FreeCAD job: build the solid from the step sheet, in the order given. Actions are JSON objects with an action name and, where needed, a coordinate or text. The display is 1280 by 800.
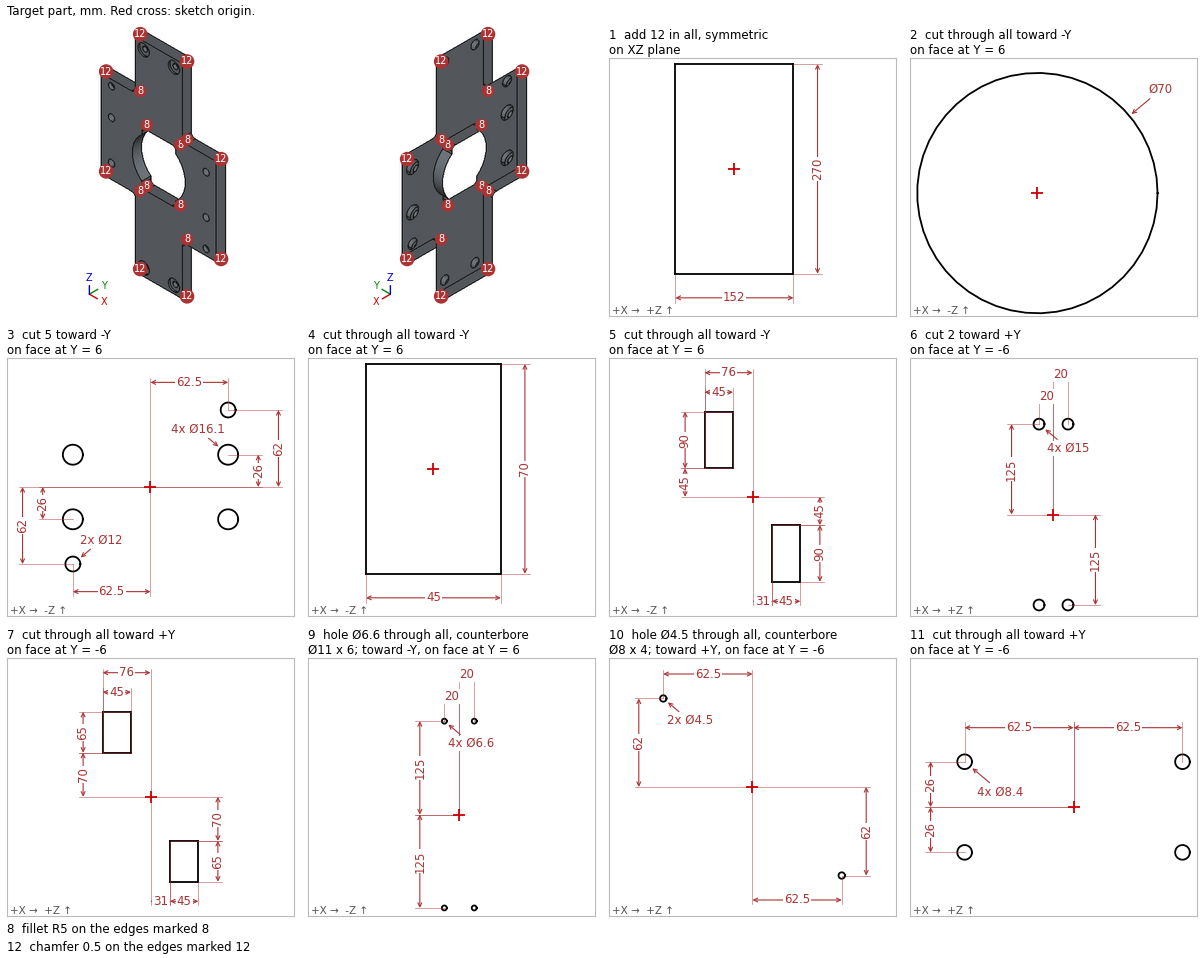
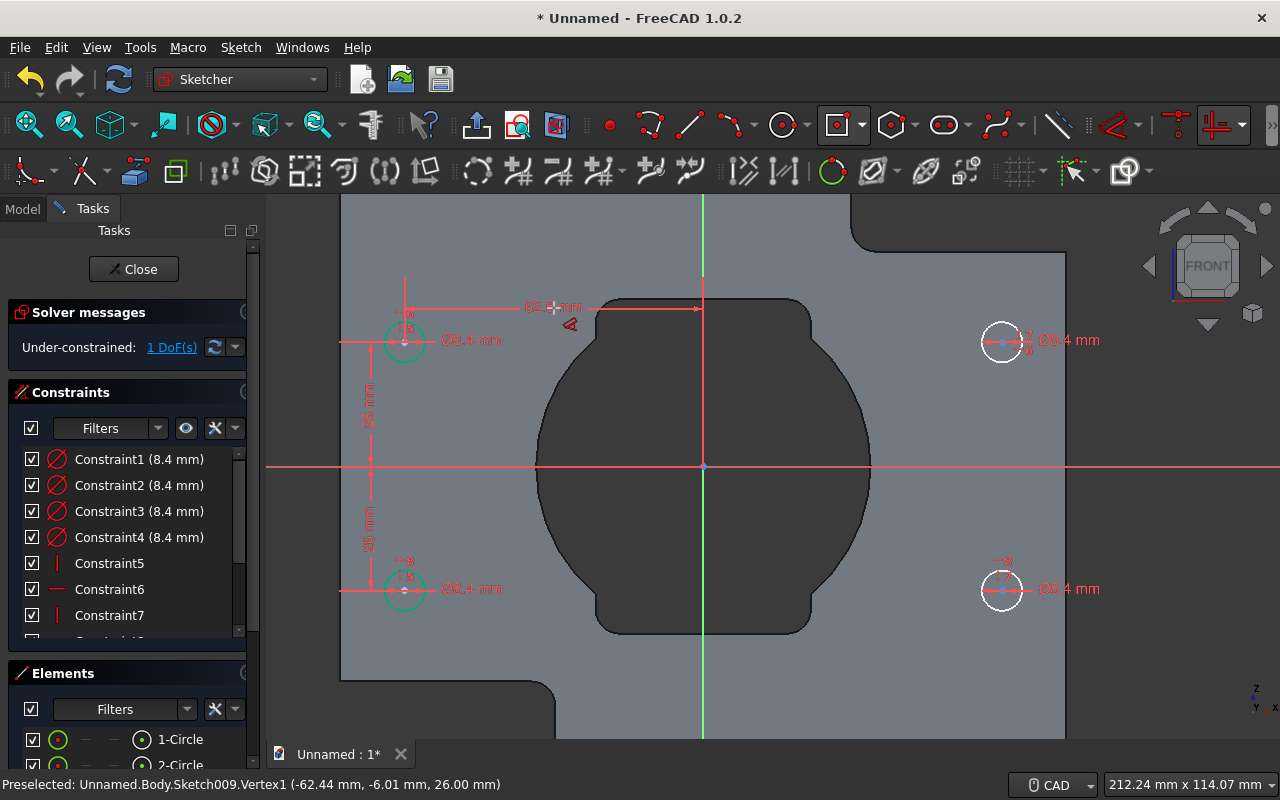
{"action": "left_click", "coordinate": [1002, 342]}
{"action": "left_click", "coordinate": [853, 308]}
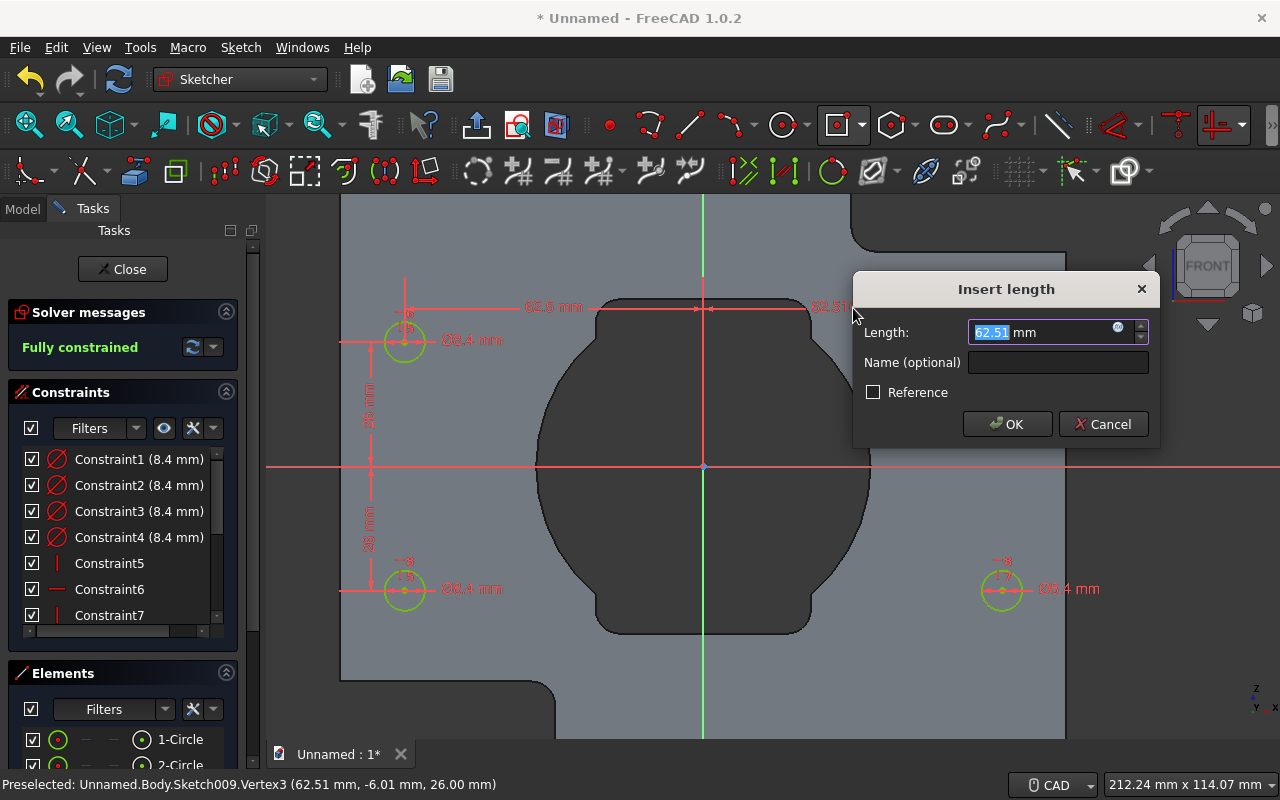
{"action": "type", "text": "62.5"}
{"action": "key", "text": "Return"}
{"action": "key", "text": "Escape"}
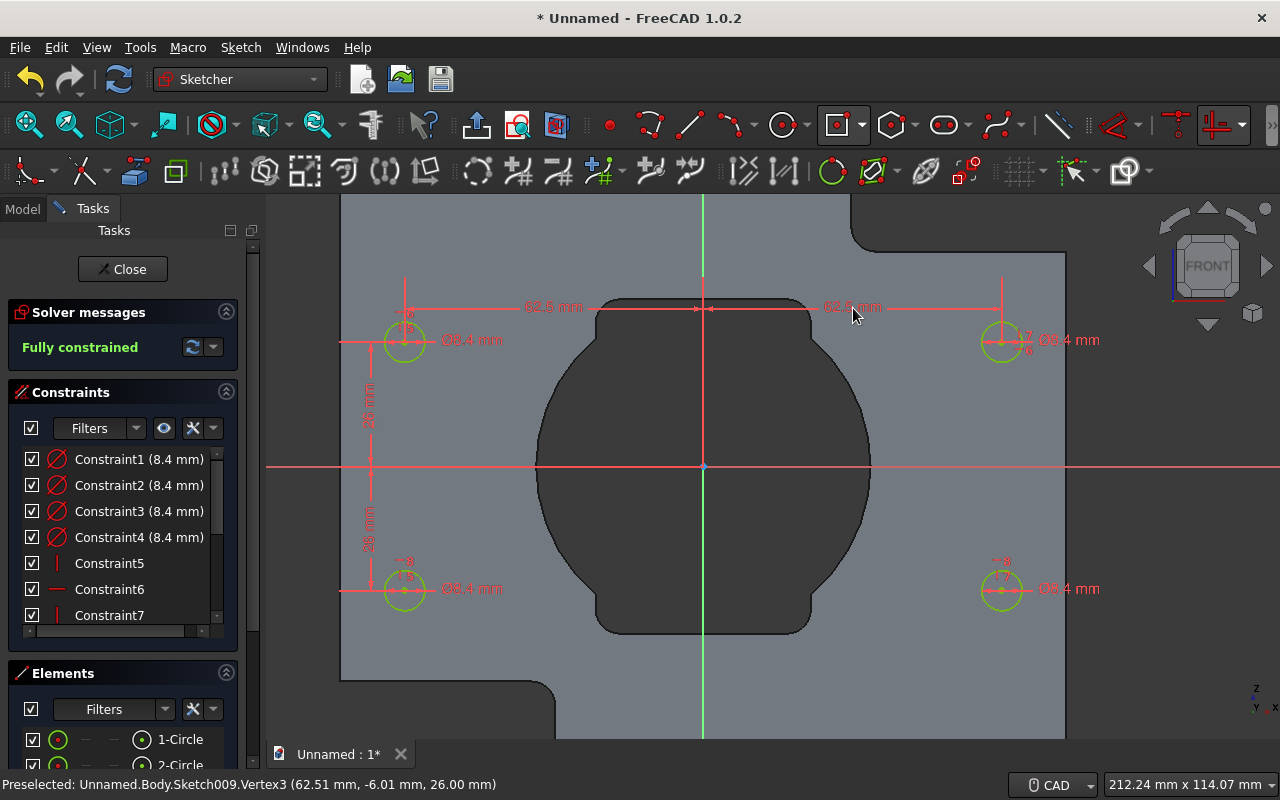
{"action": "left_click", "coordinate": [123, 269]}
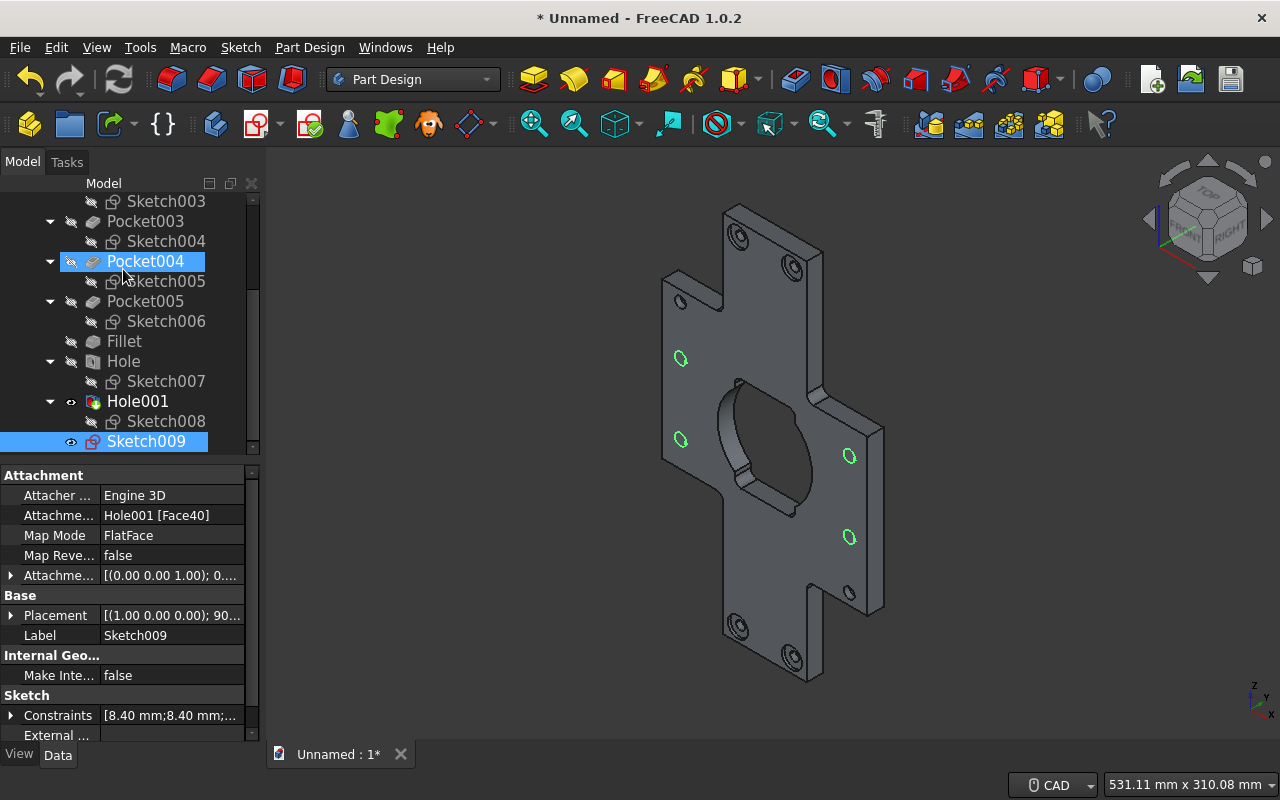
{"action": "left_click", "coordinate": [796, 80]}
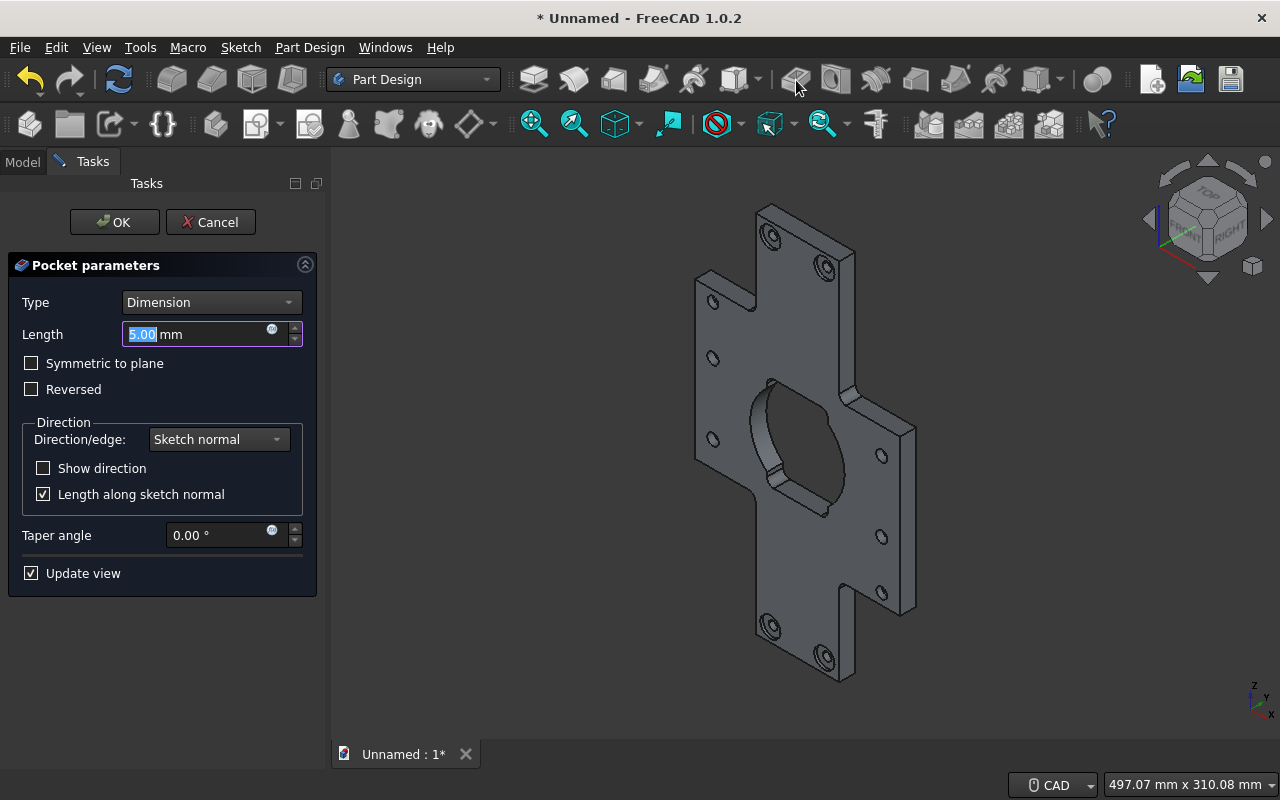
{"action": "left_click", "coordinate": [212, 302]}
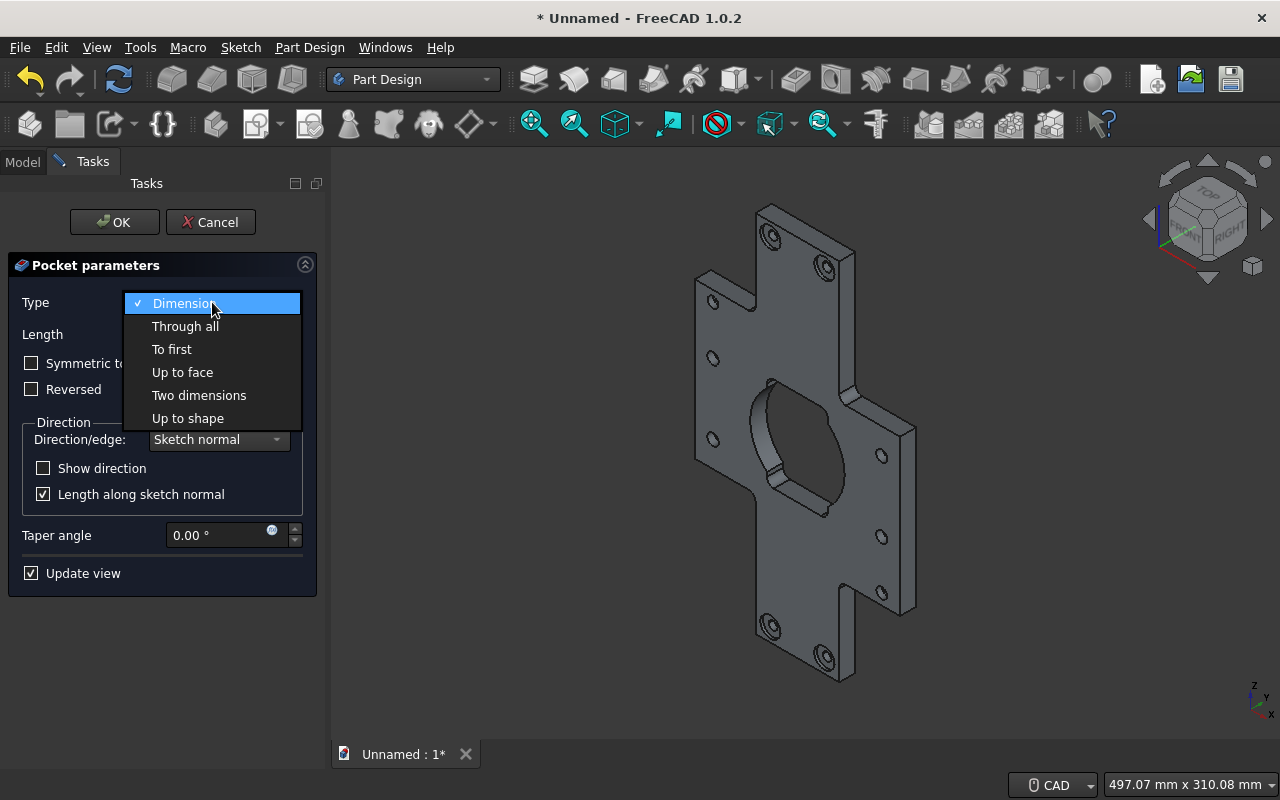
{"action": "left_click", "coordinate": [212, 326]}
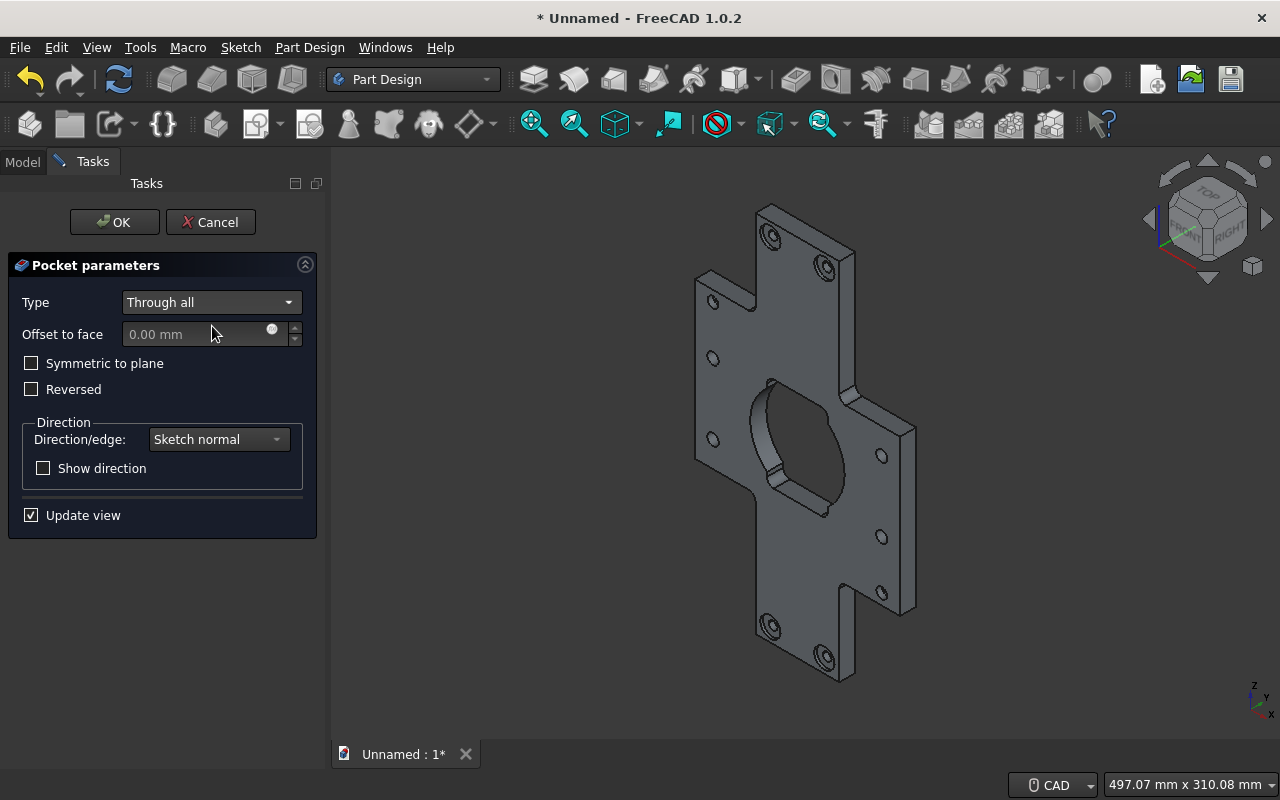
{"action": "left_click", "coordinate": [115, 222]}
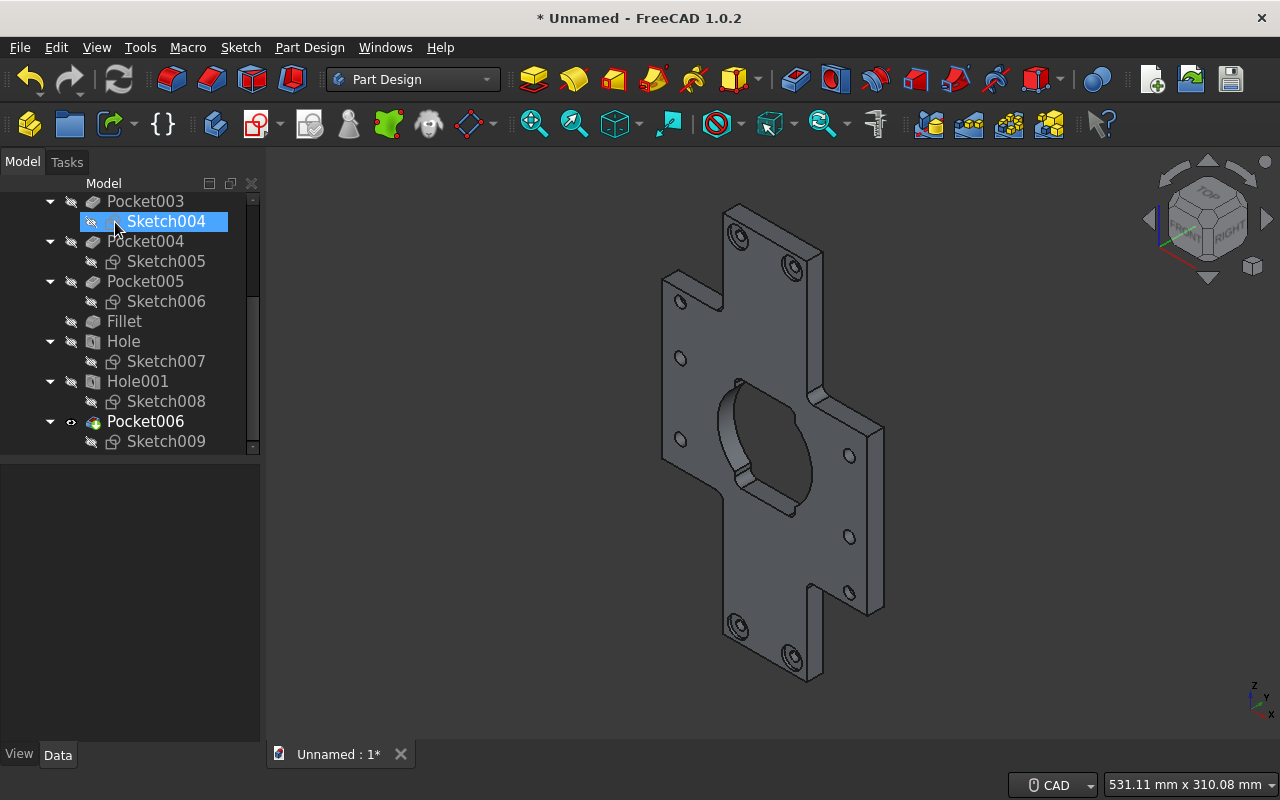
{"action": "left_click", "coordinate": [876, 431]}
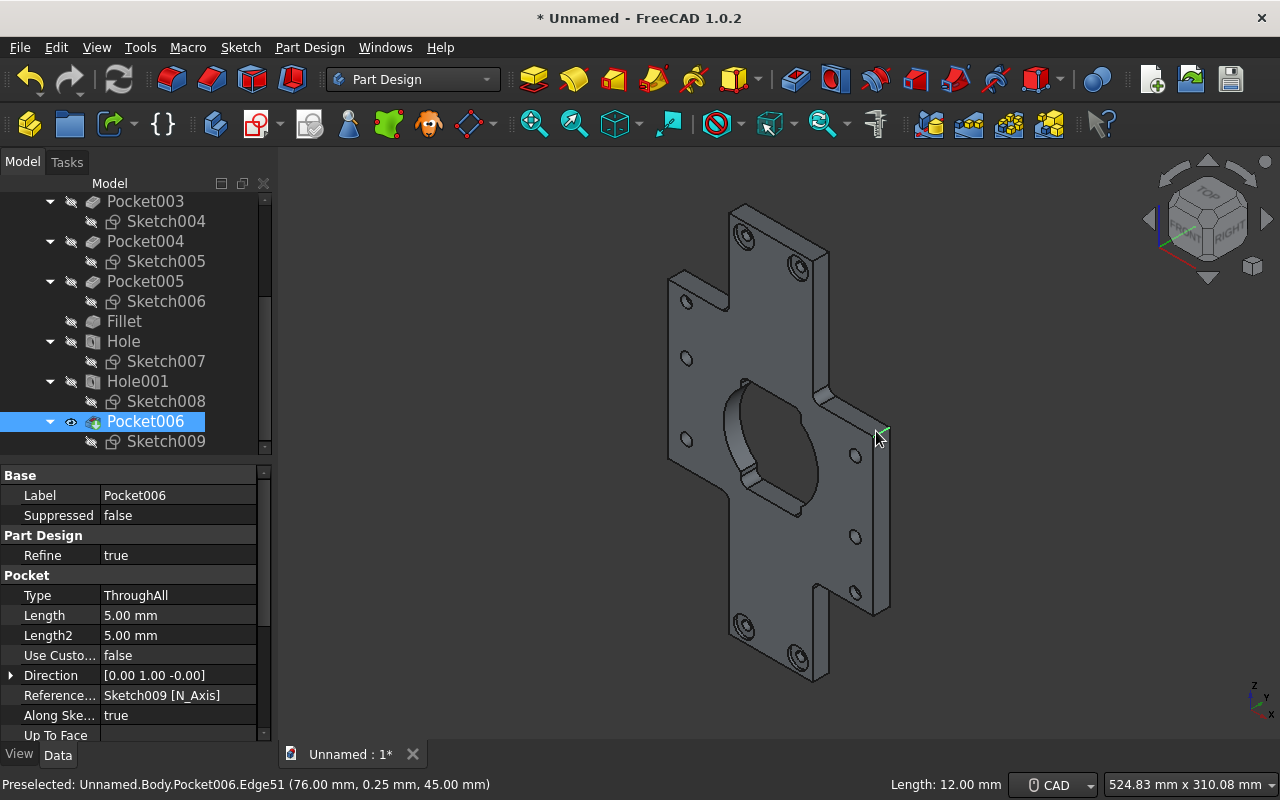
{"action": "left_click", "coordinate": [821, 256], "text": "ctrl"}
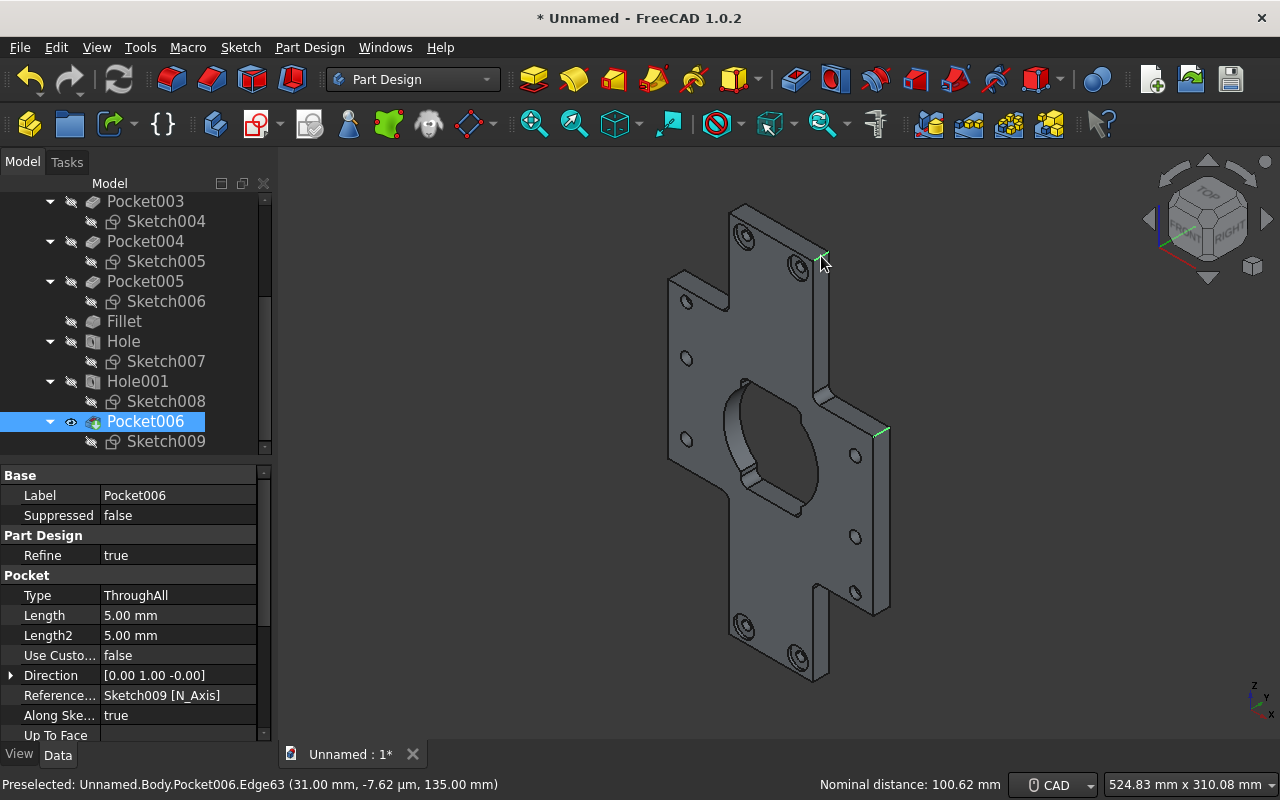
{"action": "key", "text": "2"}